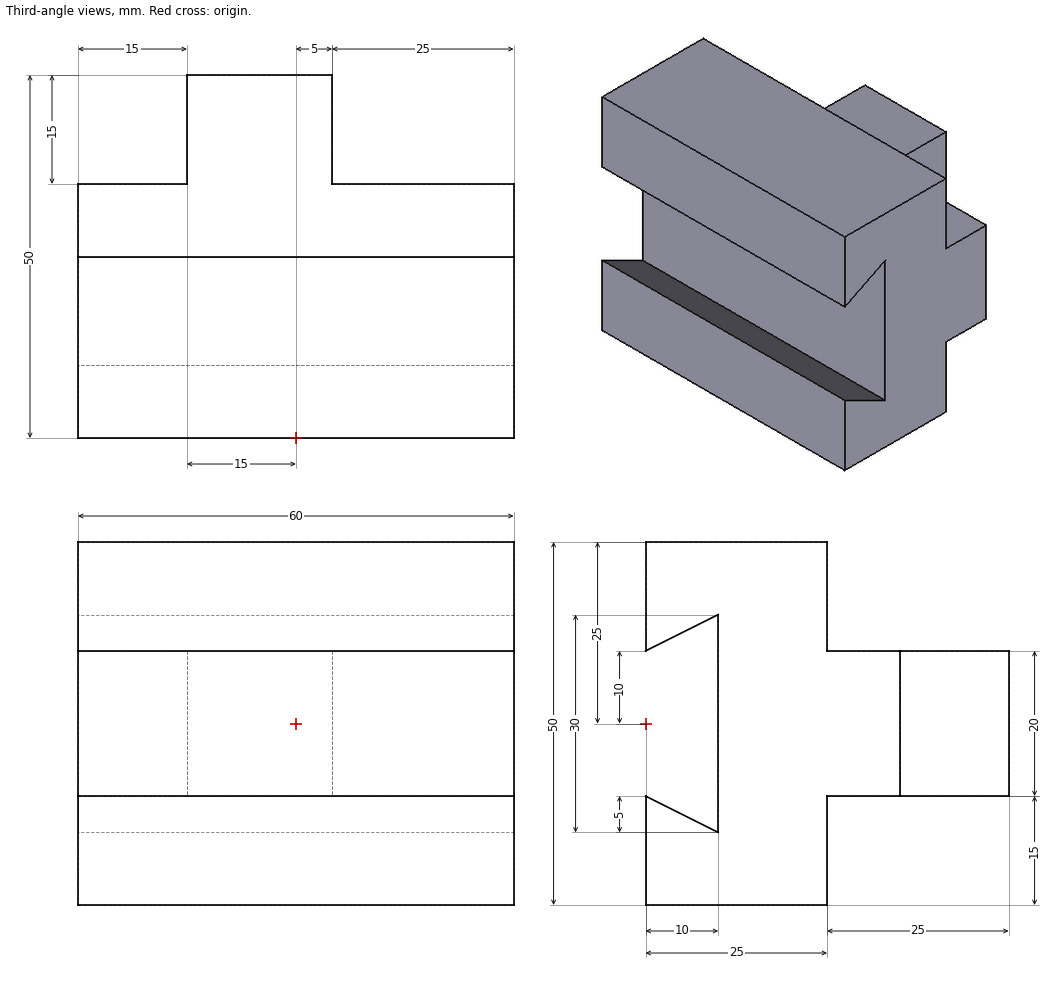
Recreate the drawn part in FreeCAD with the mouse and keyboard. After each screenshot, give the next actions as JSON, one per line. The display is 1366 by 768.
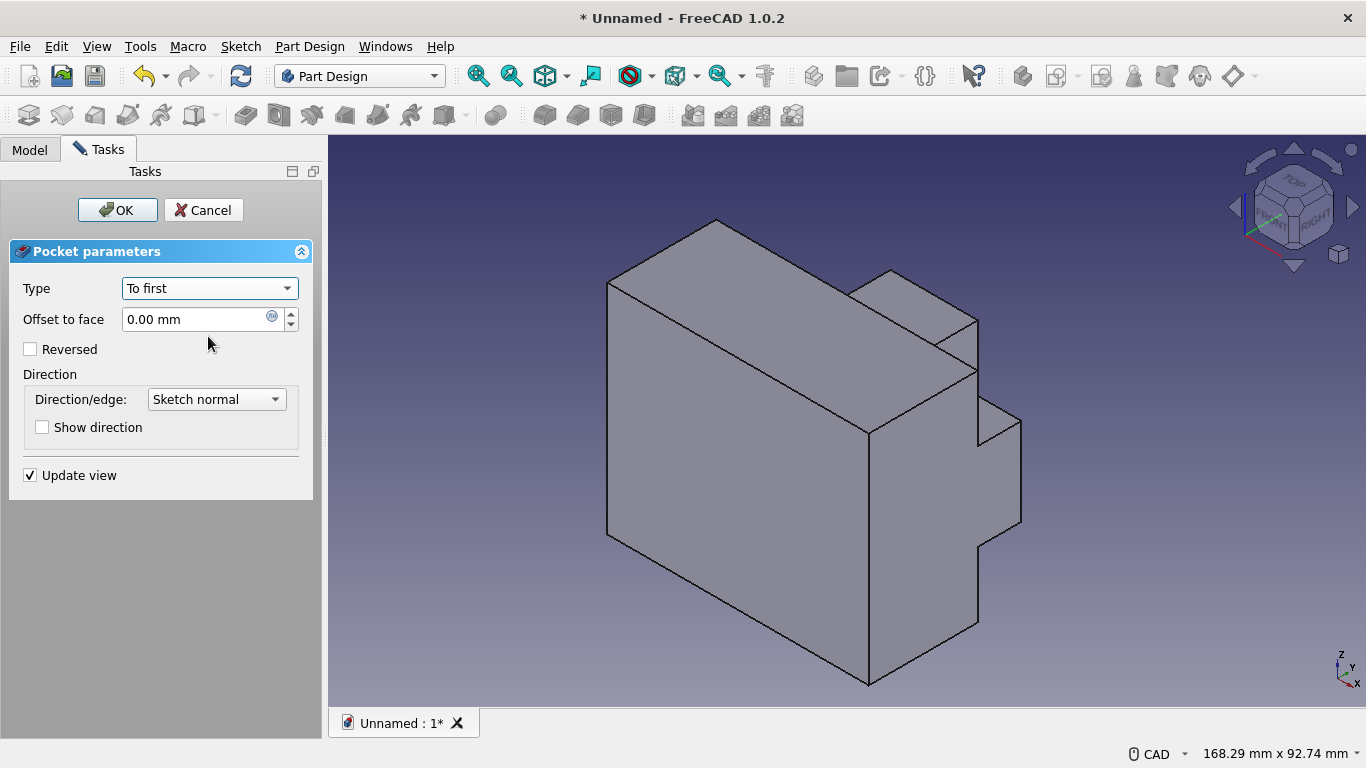
{"action": "left_click", "coordinate": [118, 210]}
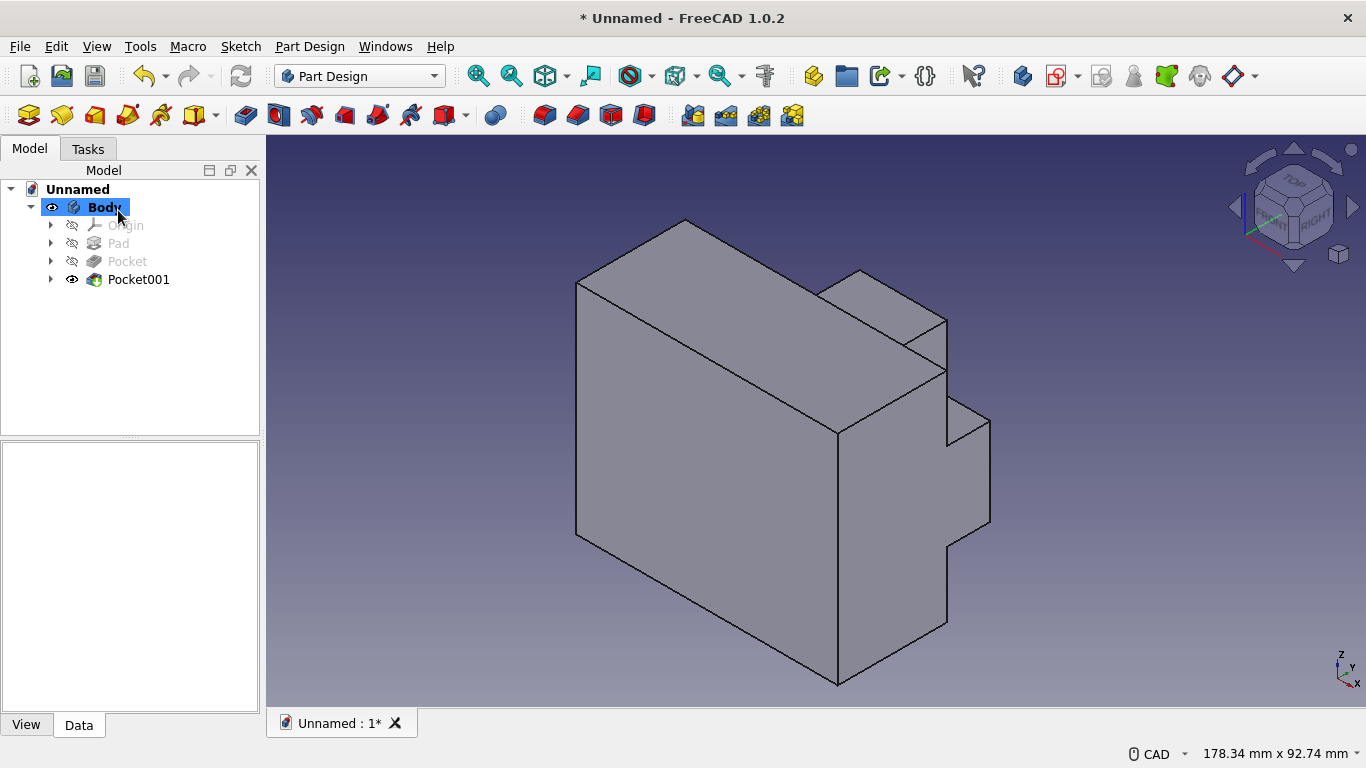
{"action": "left_click", "coordinate": [892, 563]}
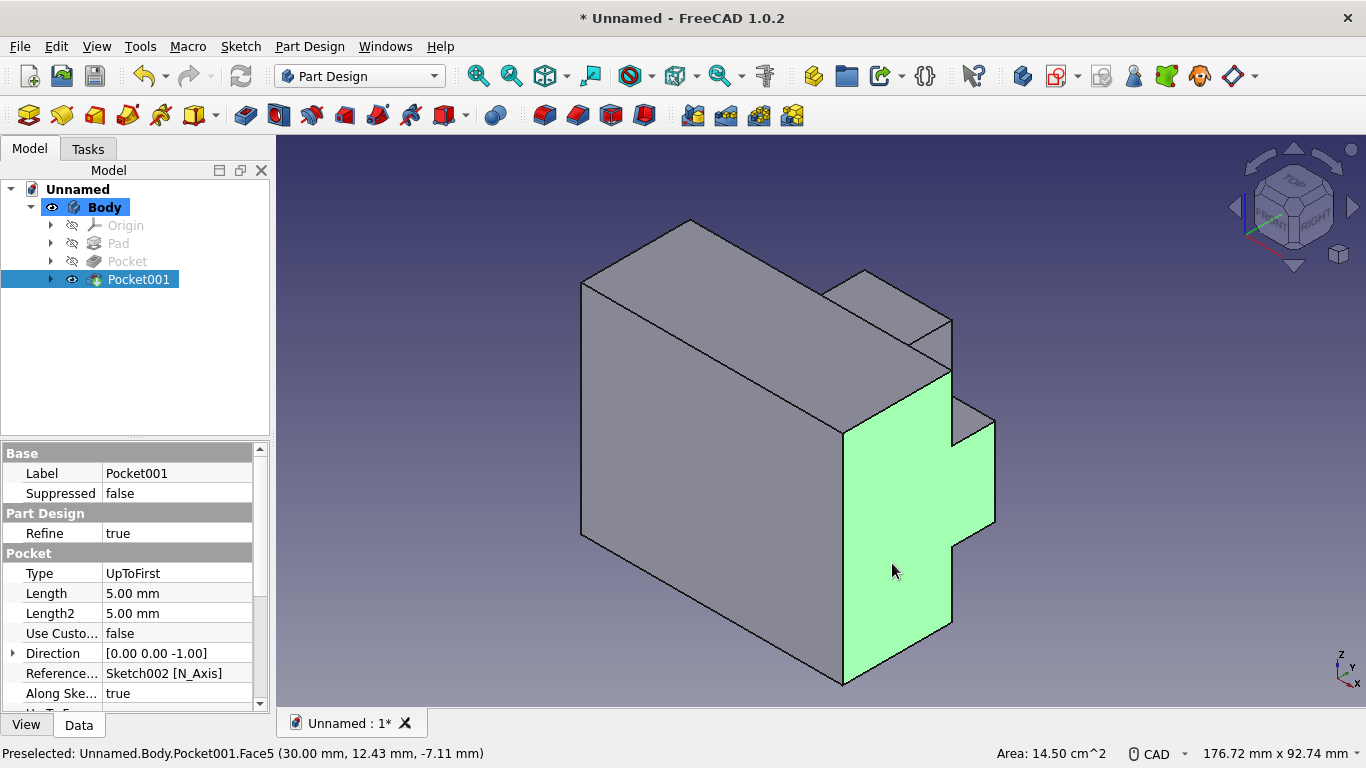
{"action": "left_click", "coordinate": [1056, 76]}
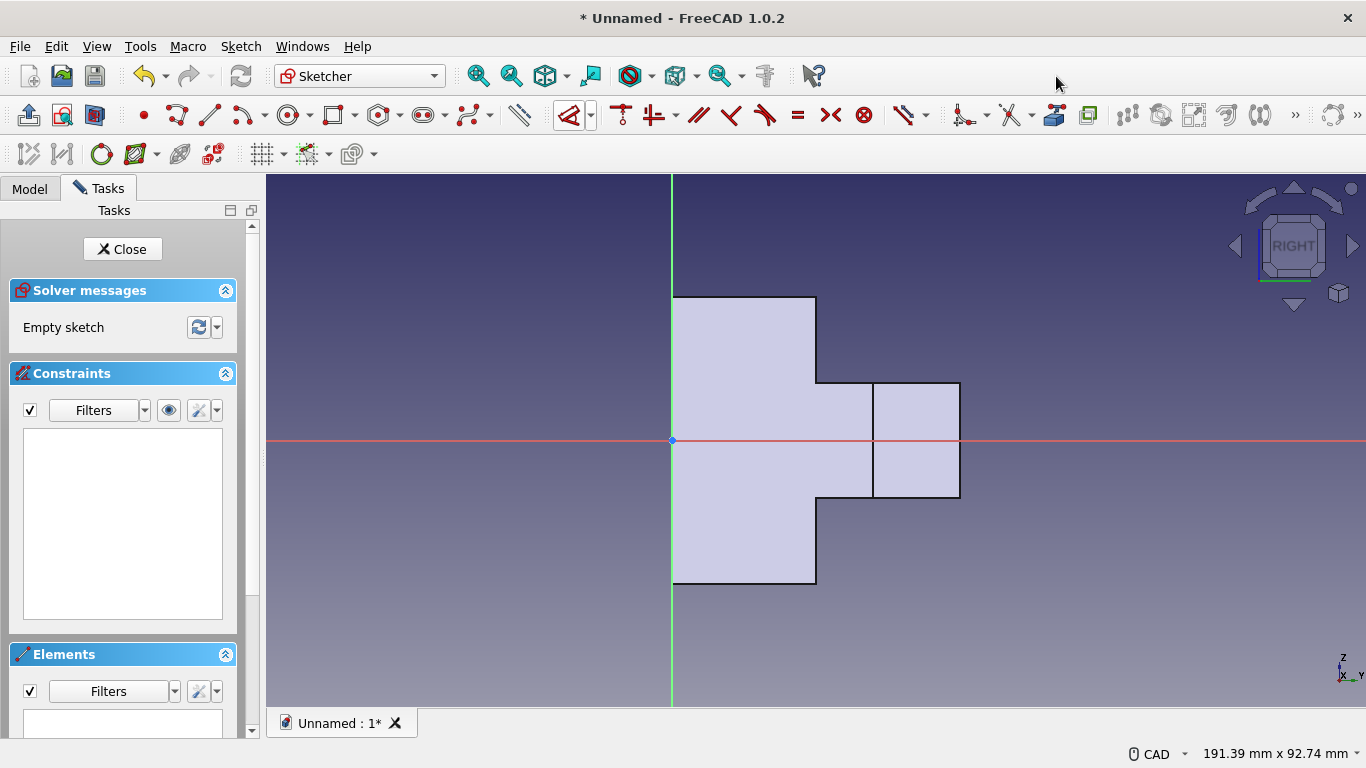
{"action": "scroll", "coordinate": [645, 440], "scroll_direction": "up", "scroll_amount": 3}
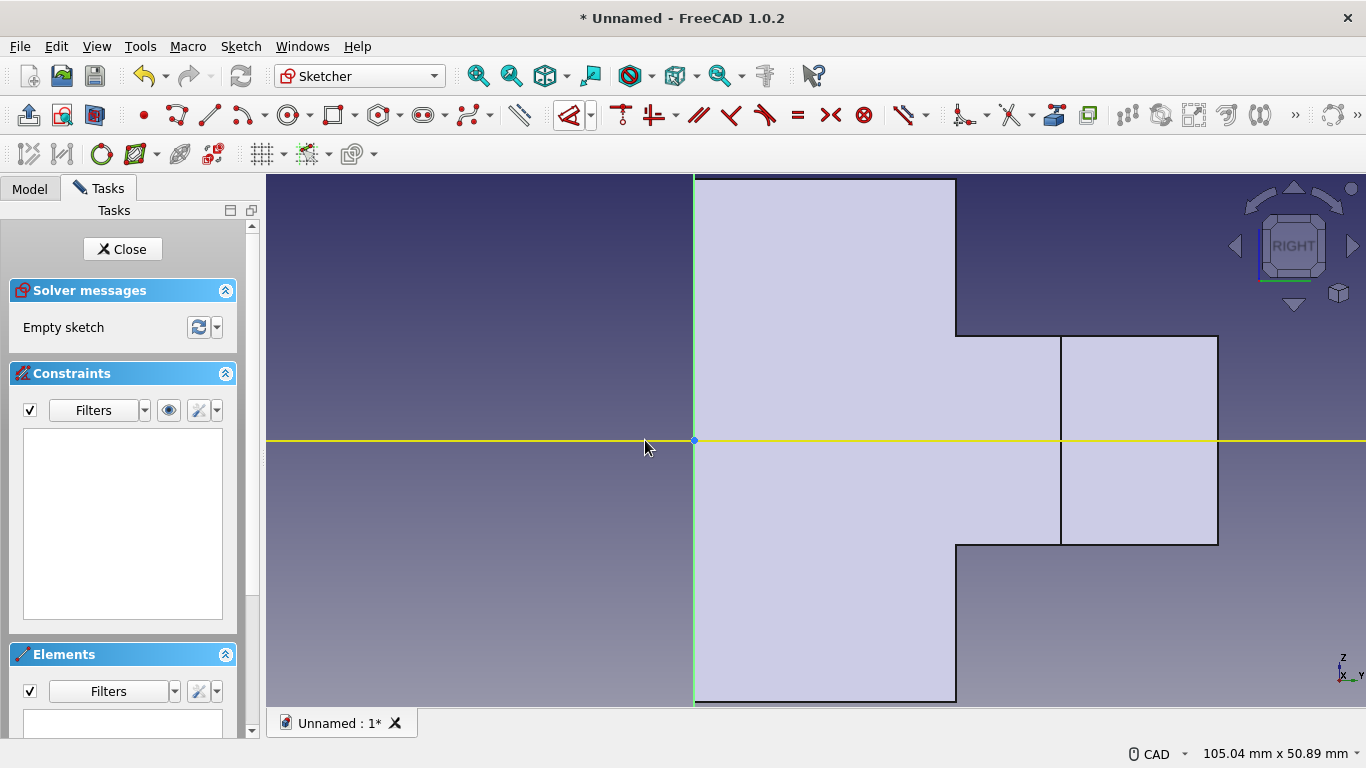
{"action": "key", "text": "g m"}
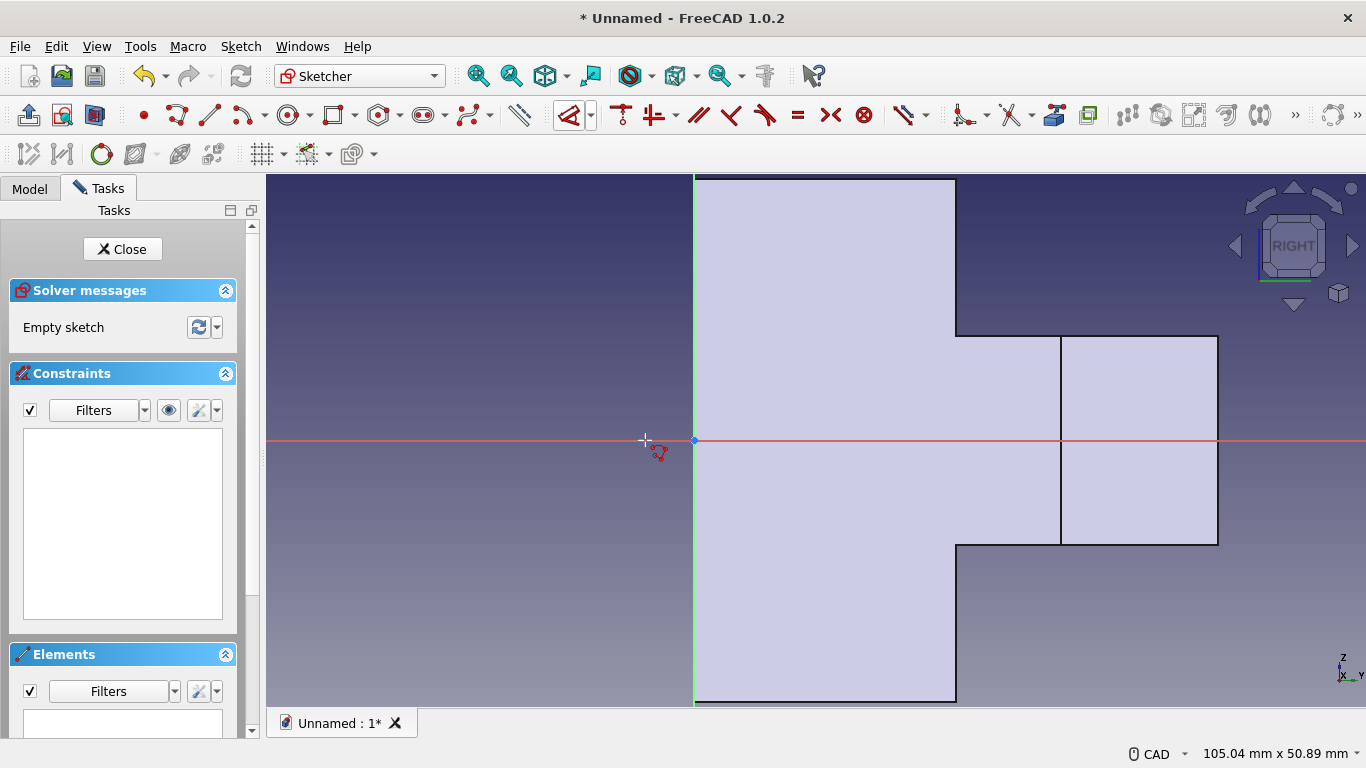
{"action": "left_click", "coordinate": [694, 336]}
{"action": "left_click", "coordinate": [703, 545]}
{"action": "left_click", "coordinate": [799, 598]}
{"action": "left_click", "coordinate": [799, 283]}
{"action": "left_click", "coordinate": [694, 337]}
{"action": "key", "text": "Escape"}
{"action": "key", "text": "Escape"}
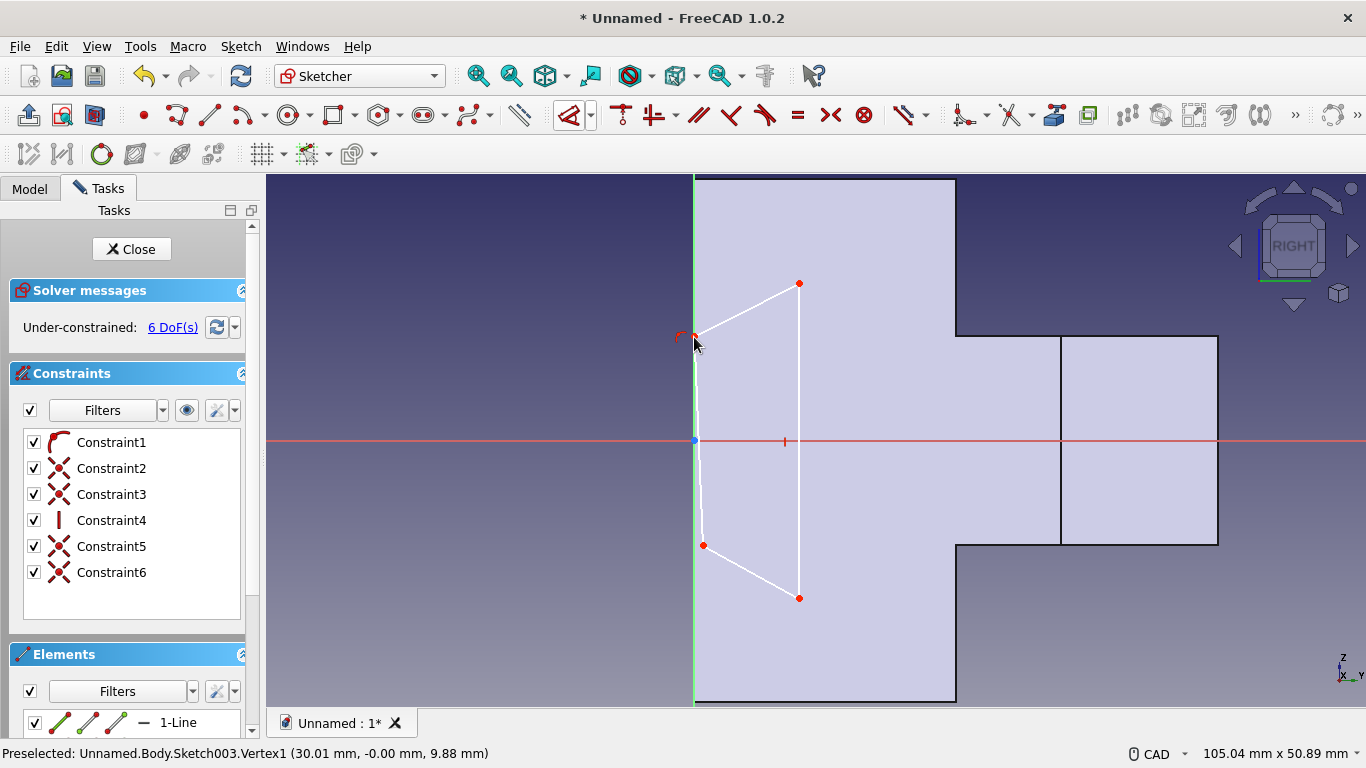
{"action": "left_click", "coordinate": [697, 400]}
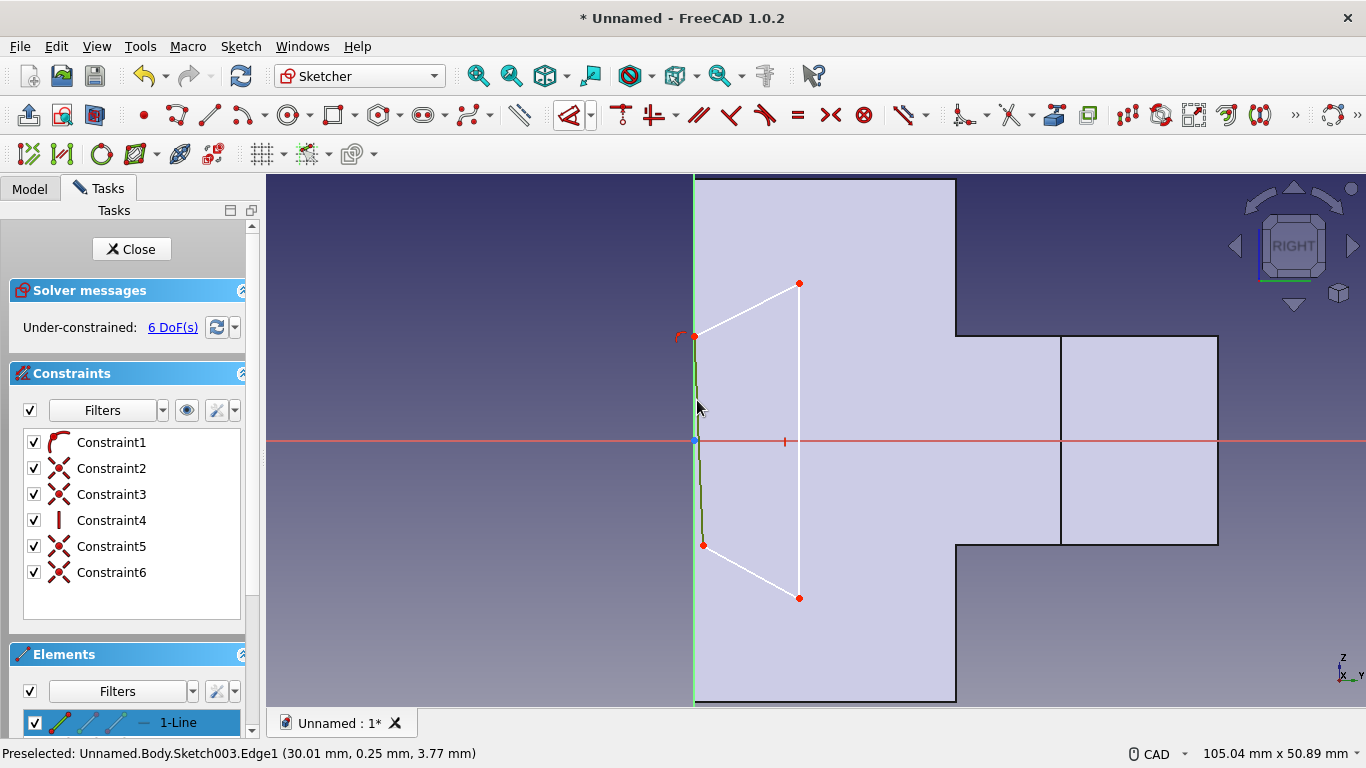
{"action": "key", "text": "v"}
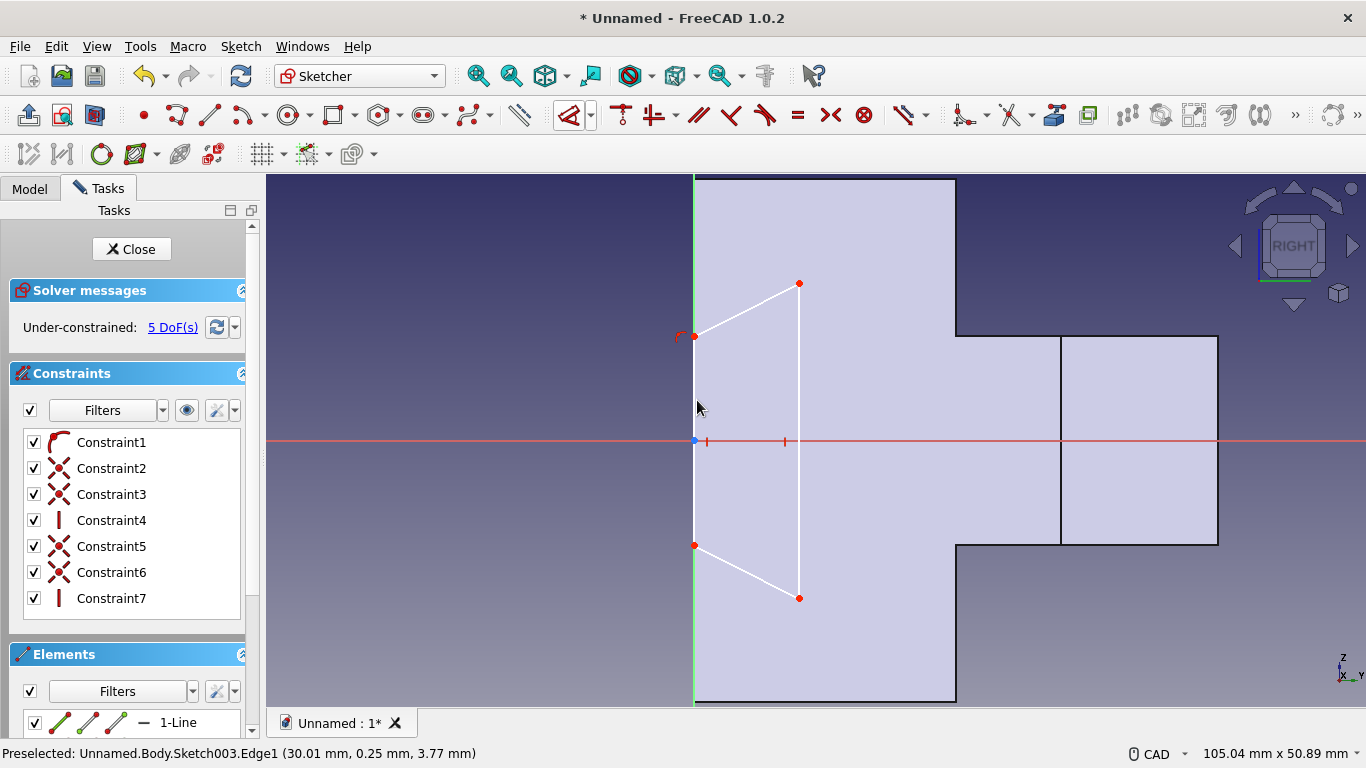
{"action": "left_click", "coordinate": [694, 400]}